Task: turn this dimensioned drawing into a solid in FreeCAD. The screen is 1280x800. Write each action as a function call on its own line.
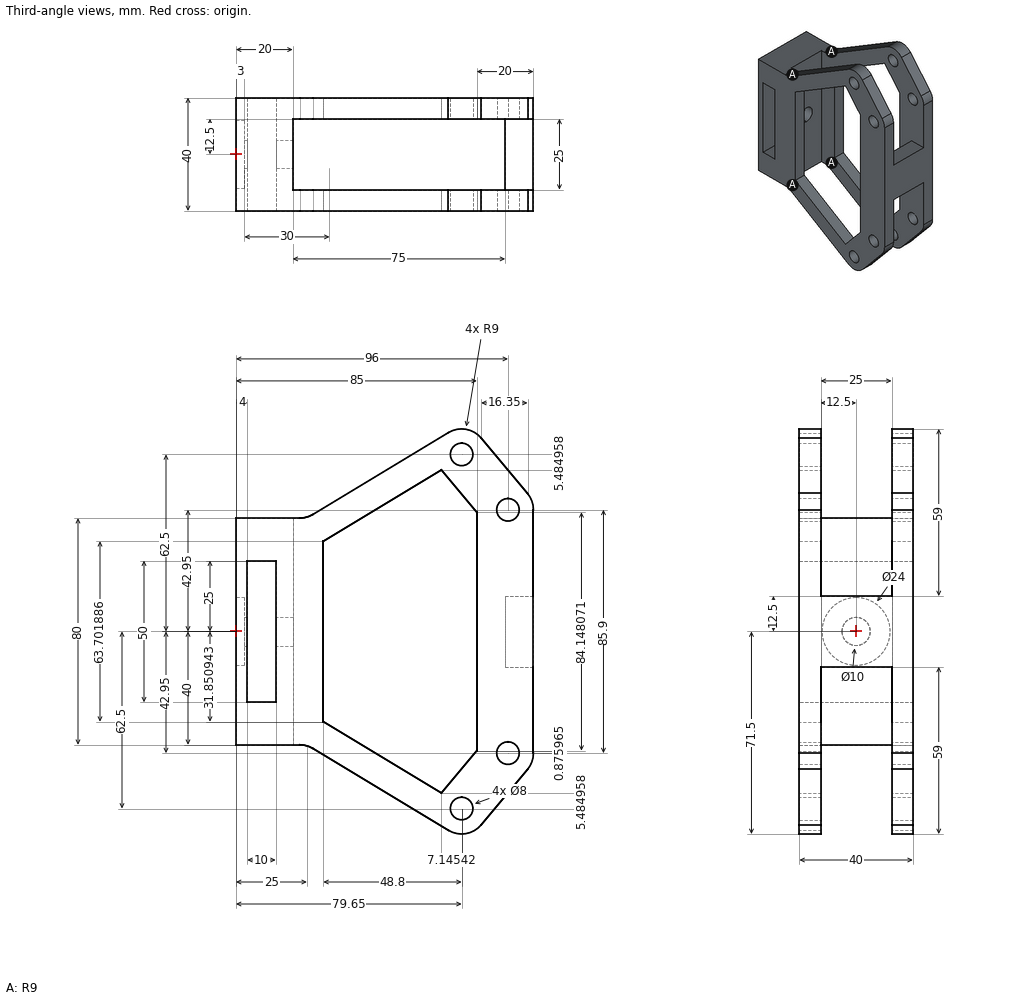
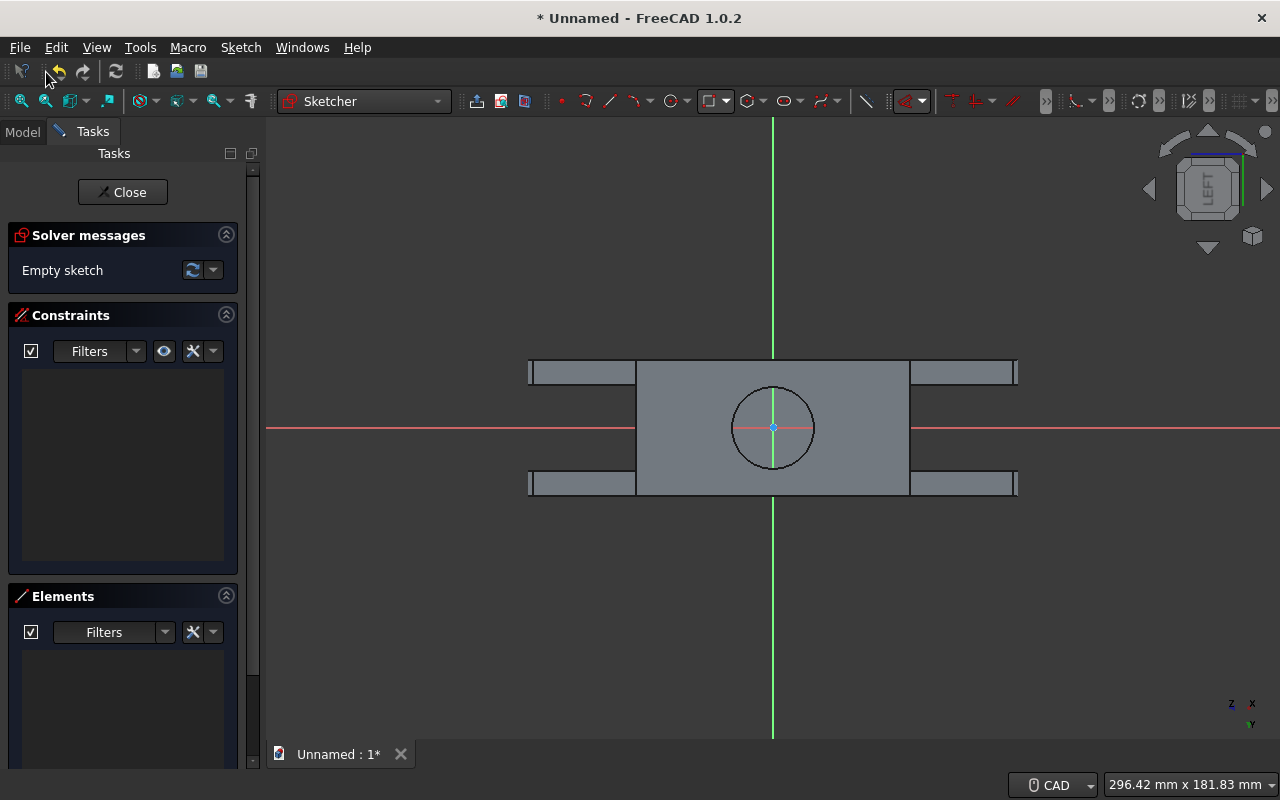
key(q)
key(s)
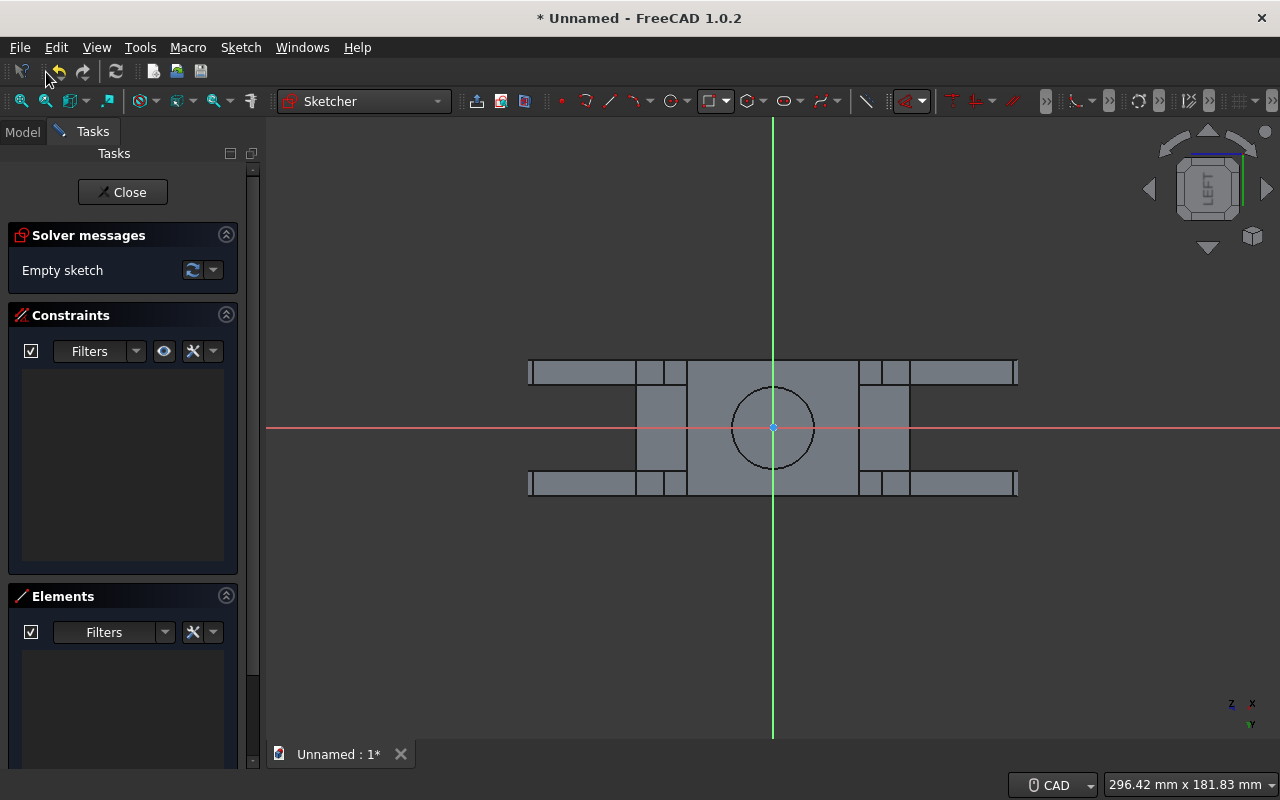
scroll(780, 428, up, 12)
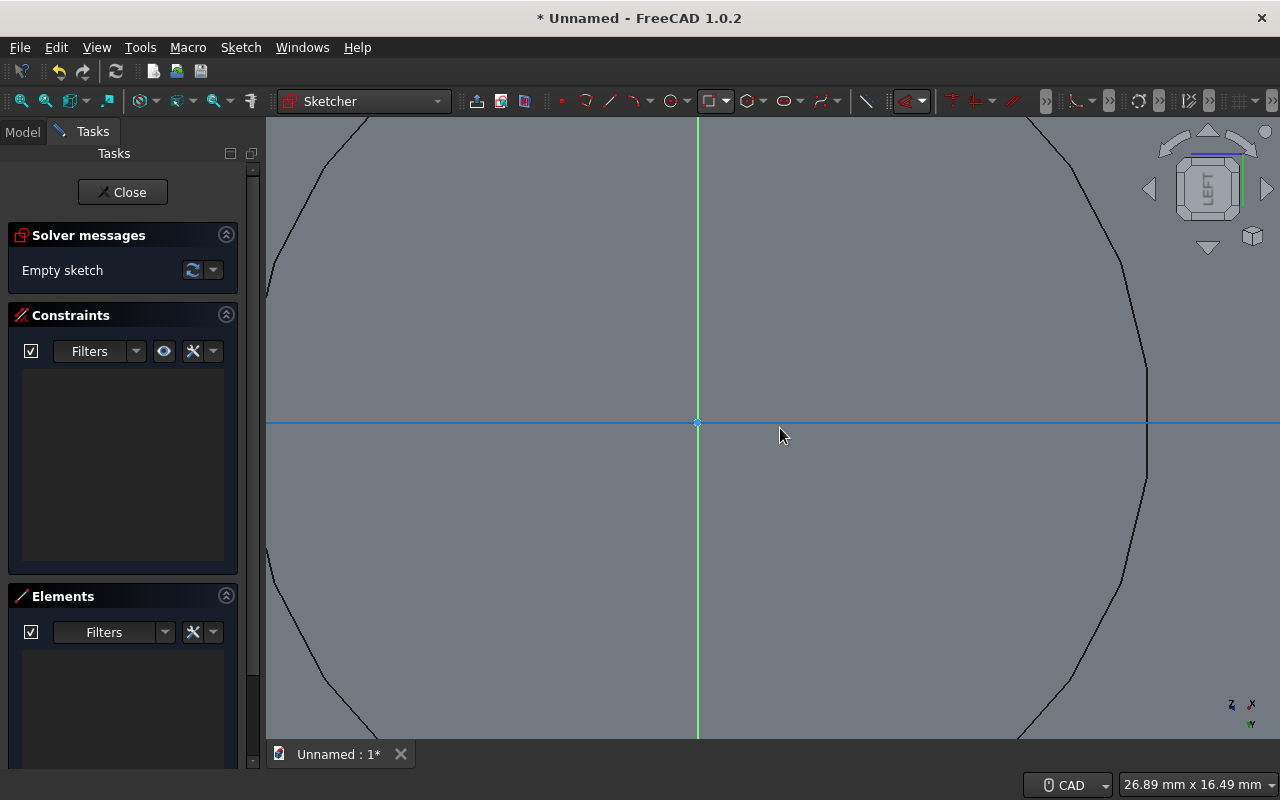
key(g)
key(c)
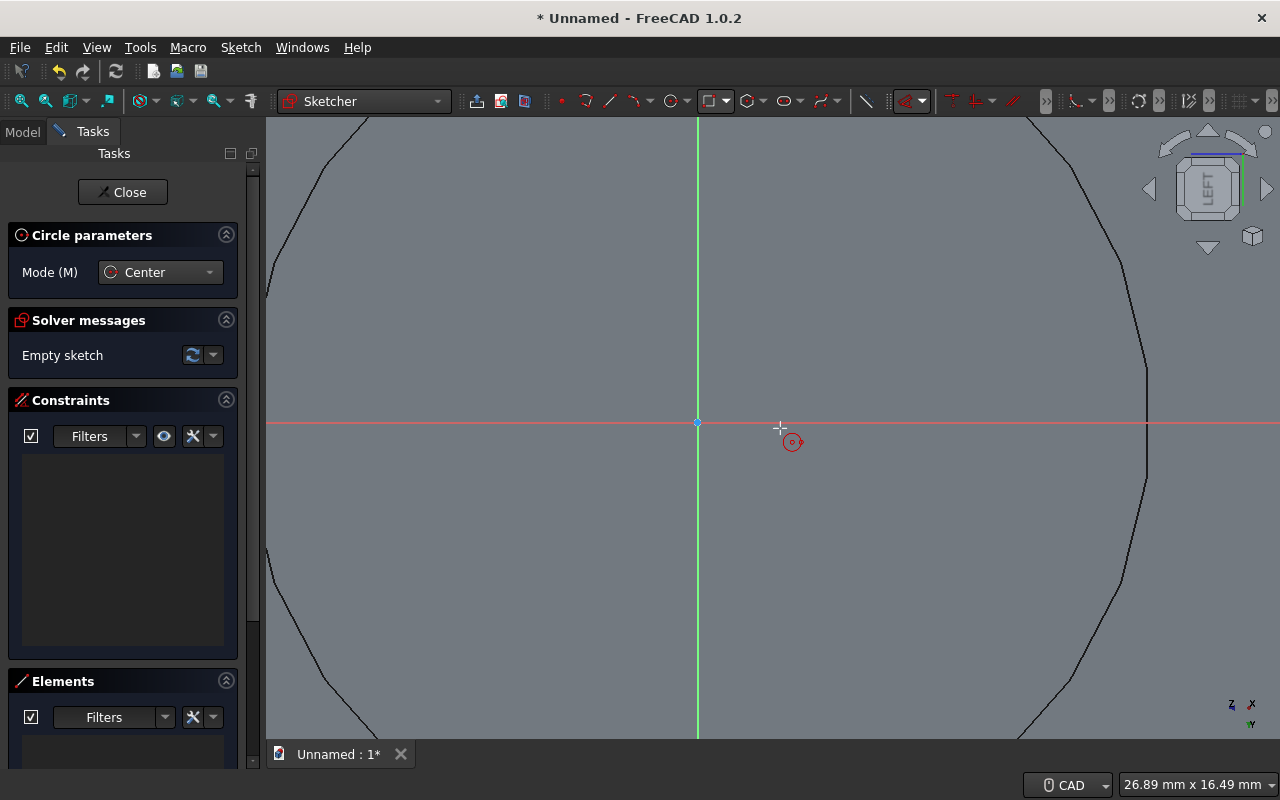
click(698, 423)
move(831, 290)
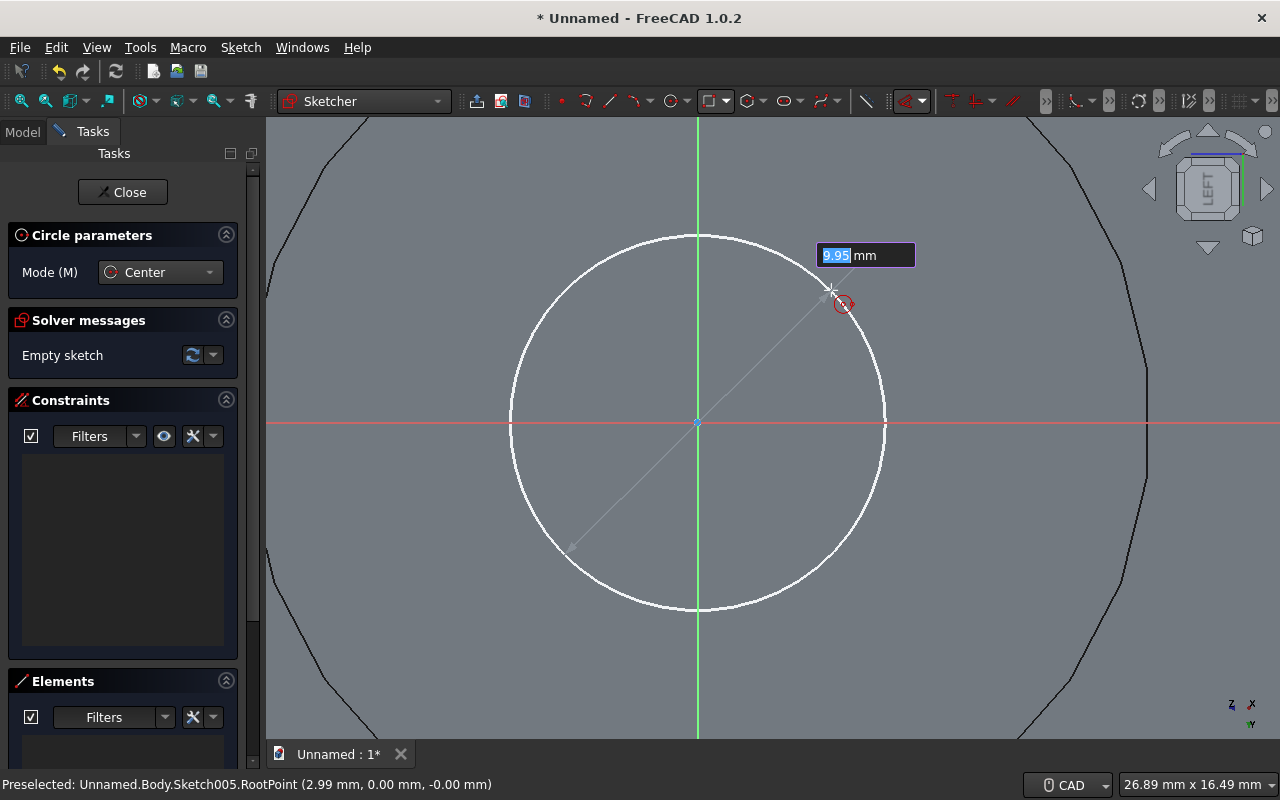
text(10)
key(Return)
key(Escape)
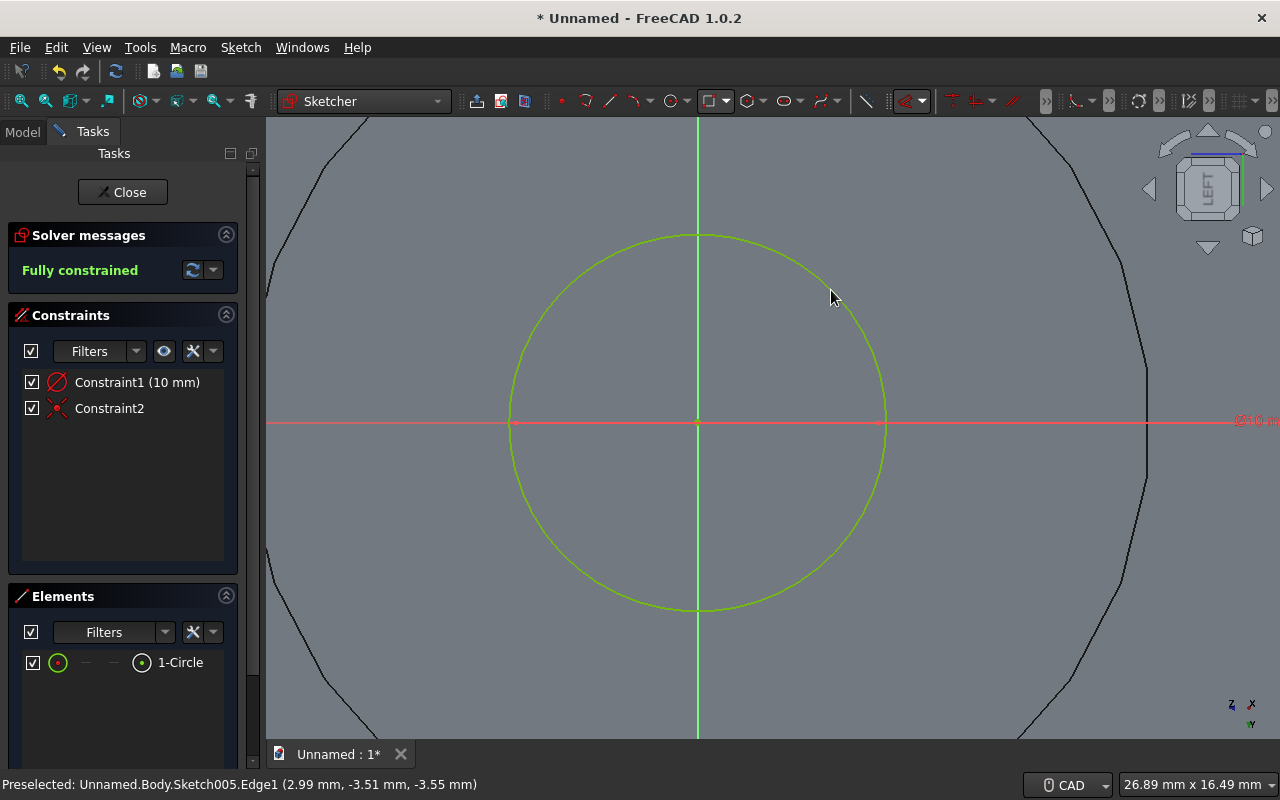
click(123, 192)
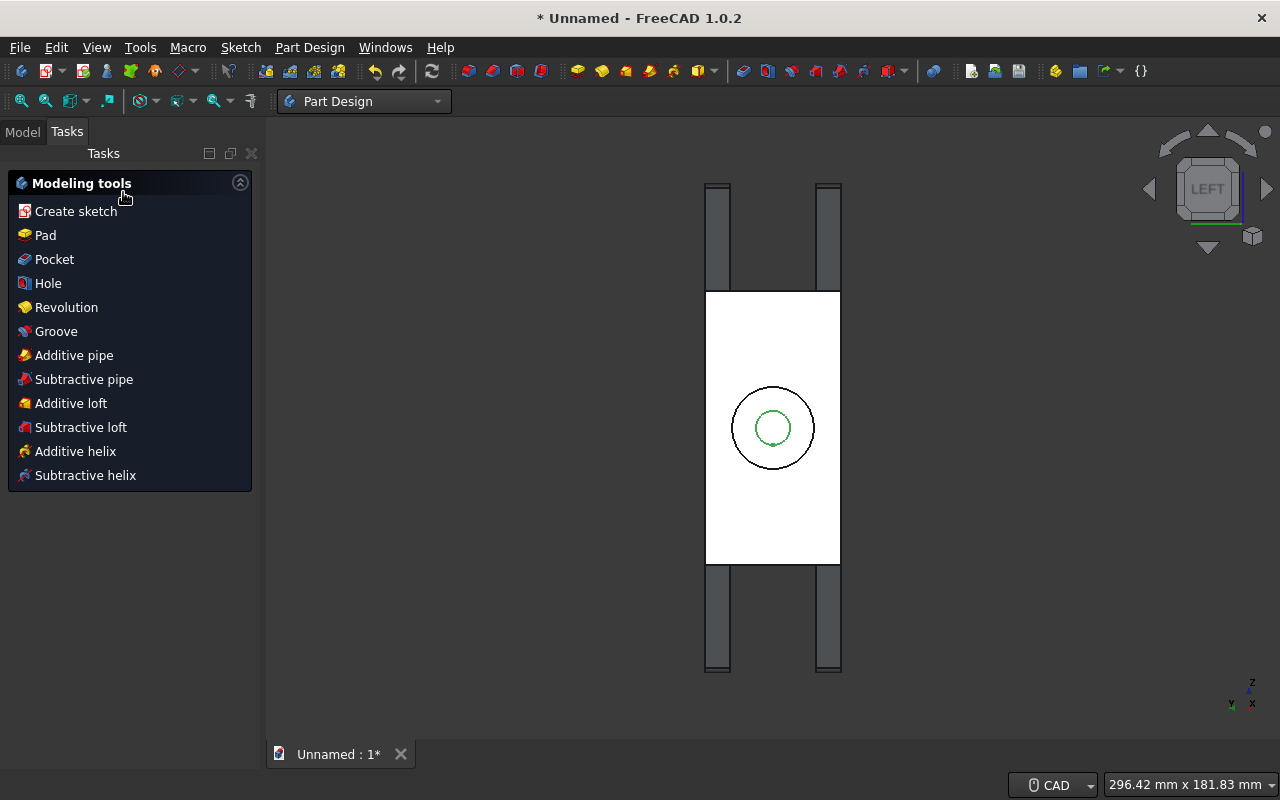
click(744, 72)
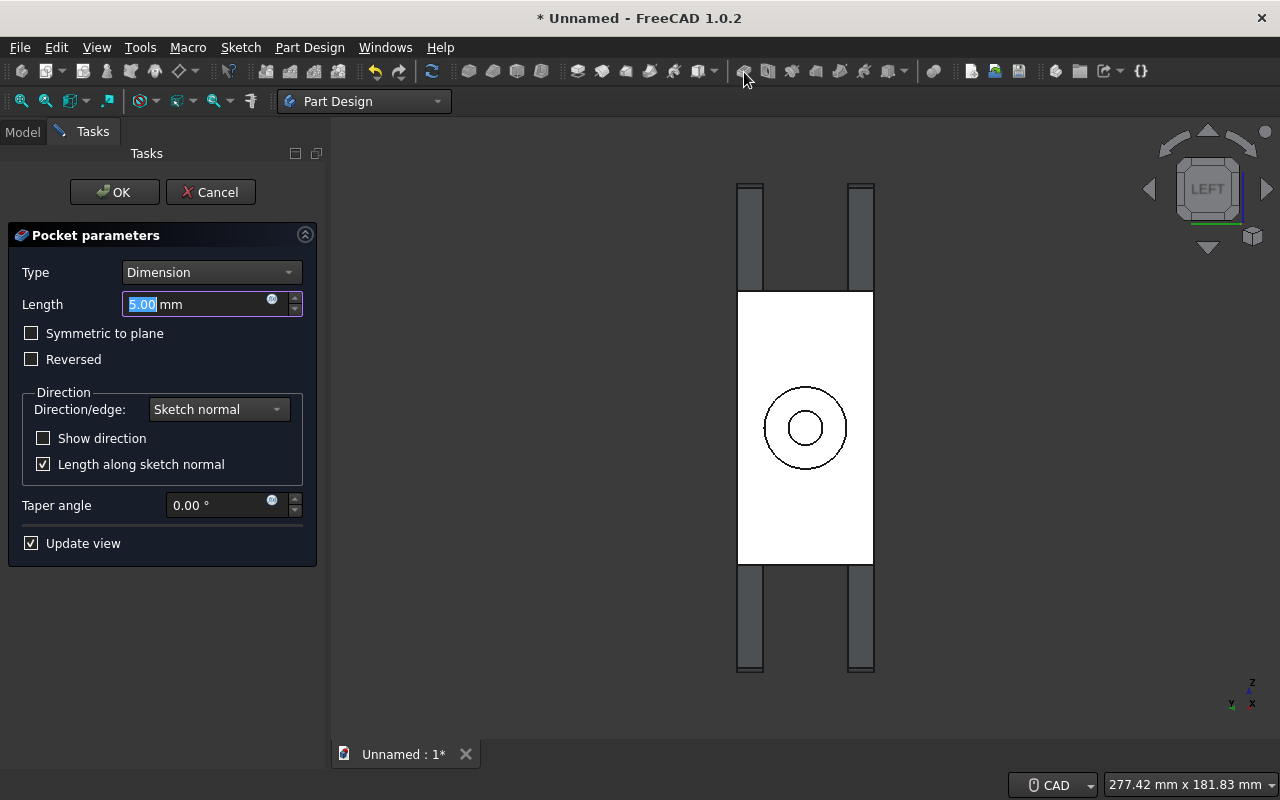
text(30)
key(Tab)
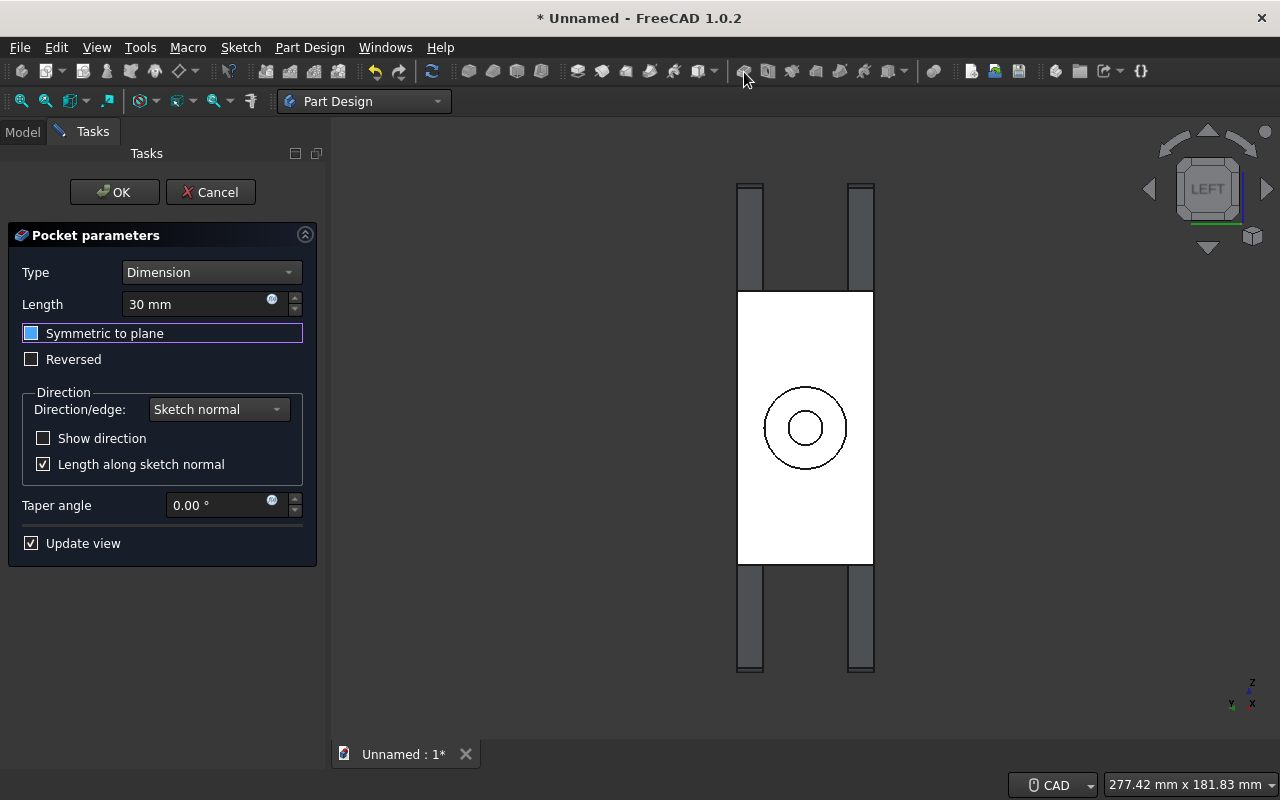
click(115, 192)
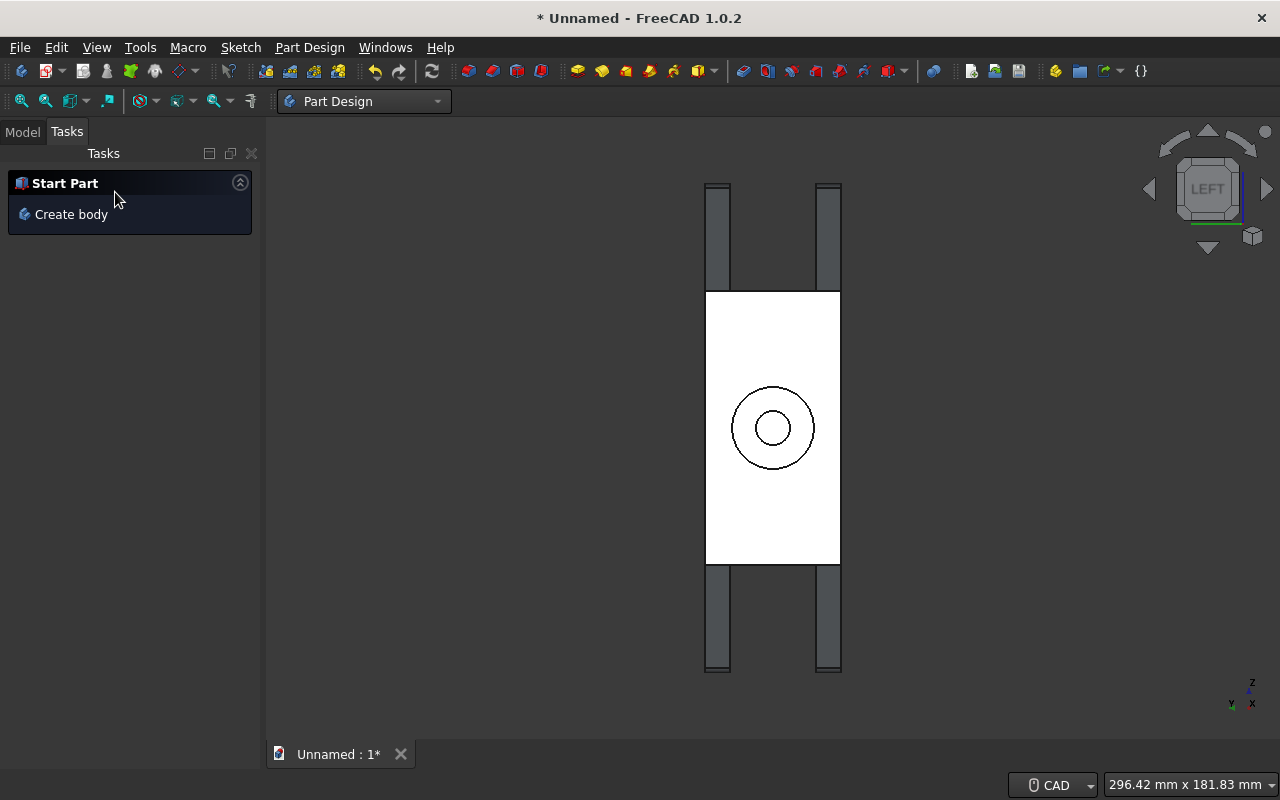
key(0)